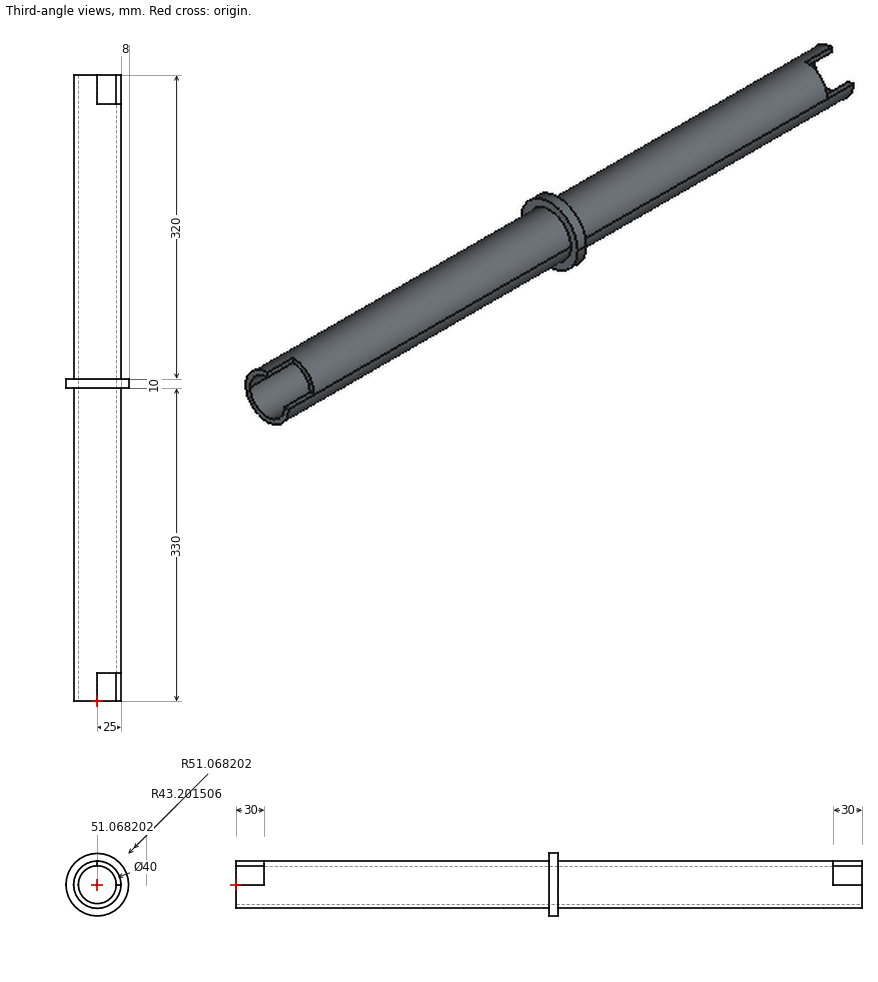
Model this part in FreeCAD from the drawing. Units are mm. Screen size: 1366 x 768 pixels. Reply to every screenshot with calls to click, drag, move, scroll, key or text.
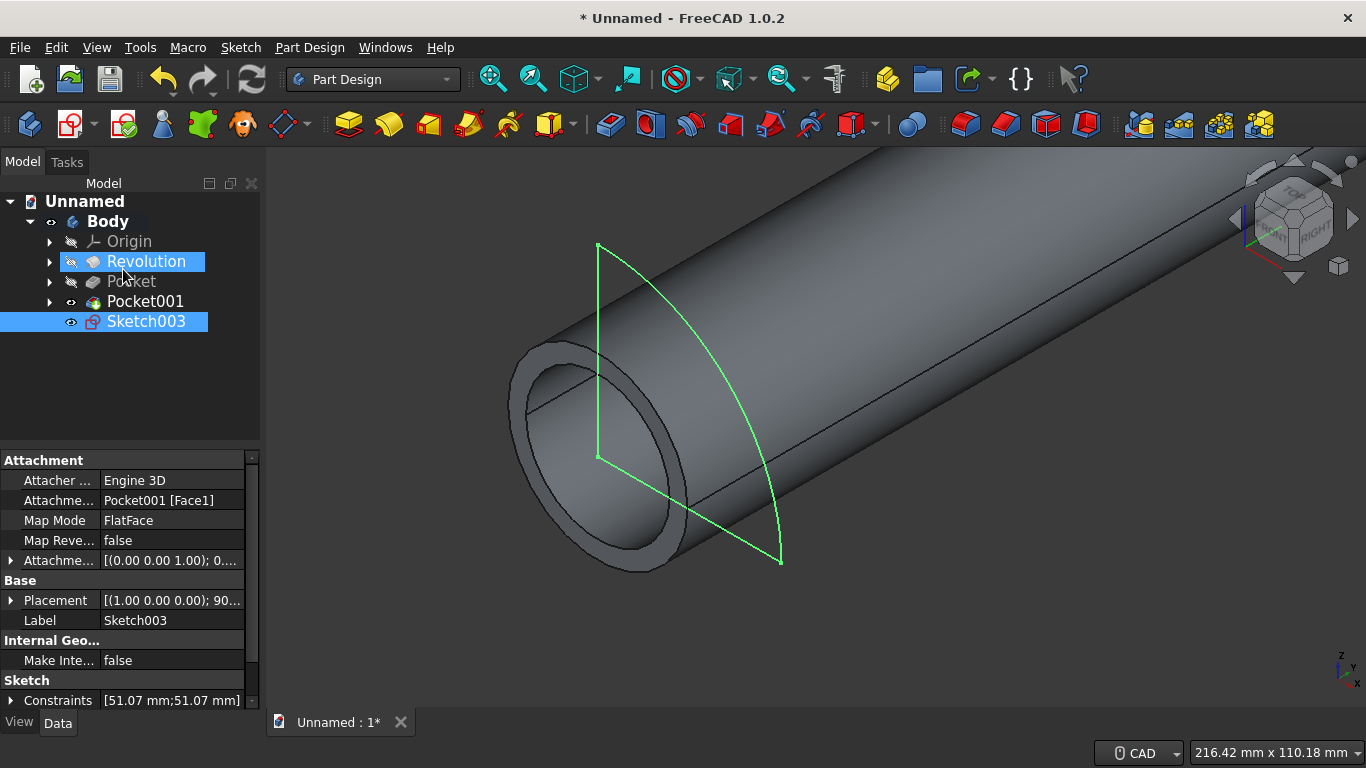
click(612, 124)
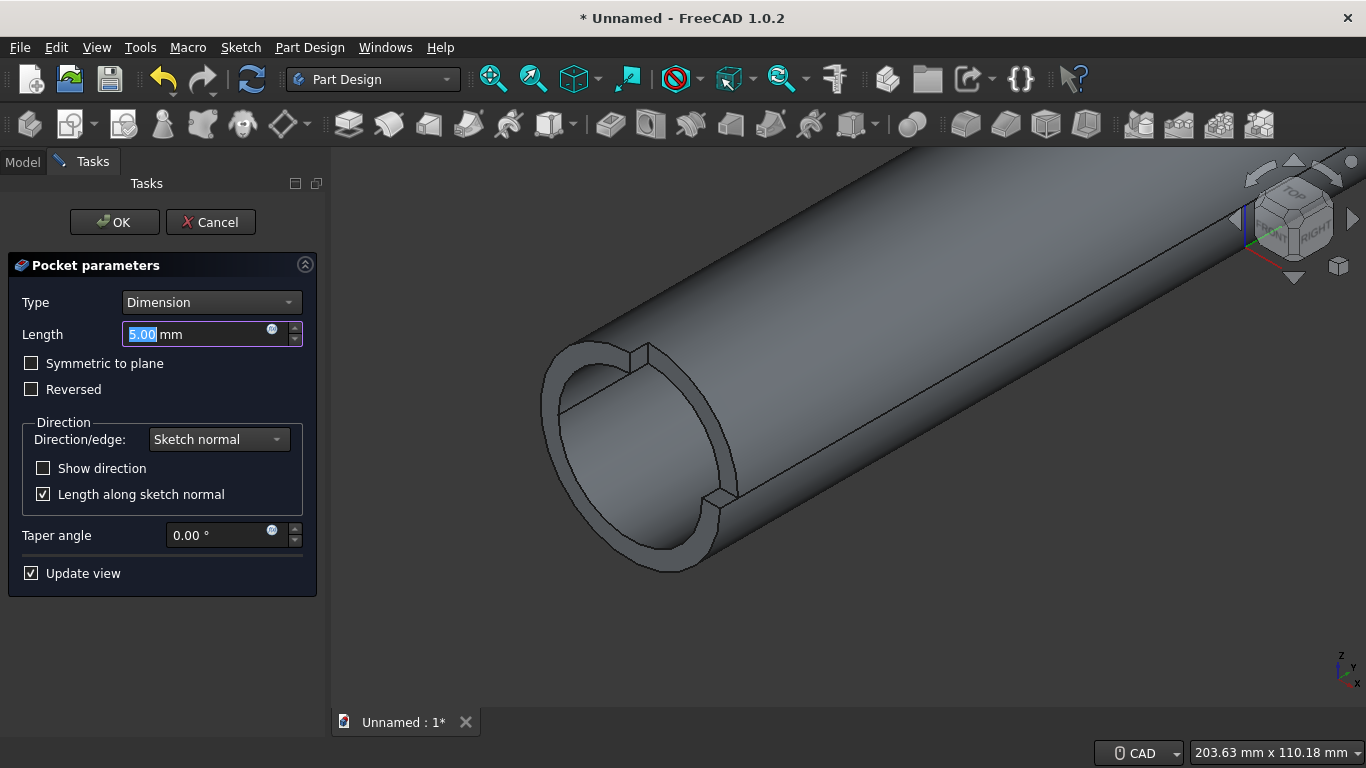
text(30)
key(Tab)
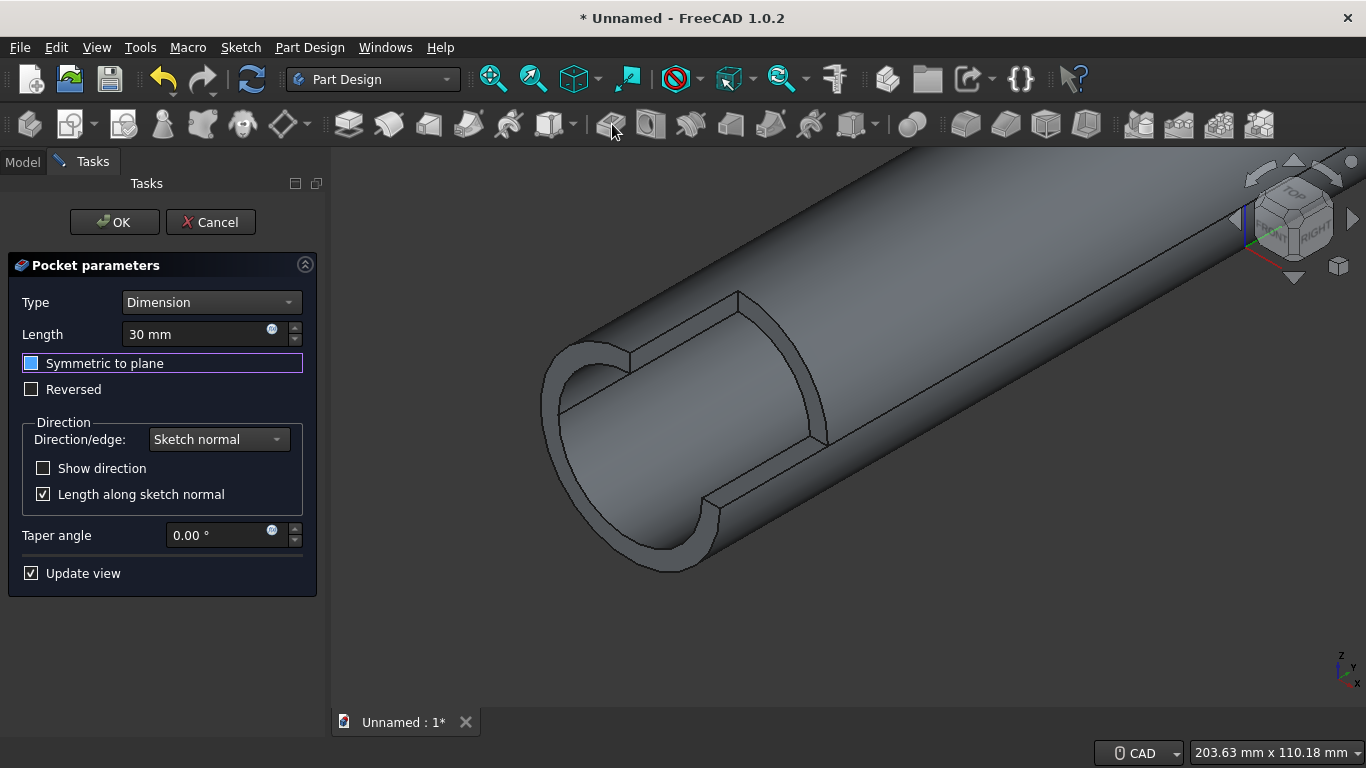
click(115, 222)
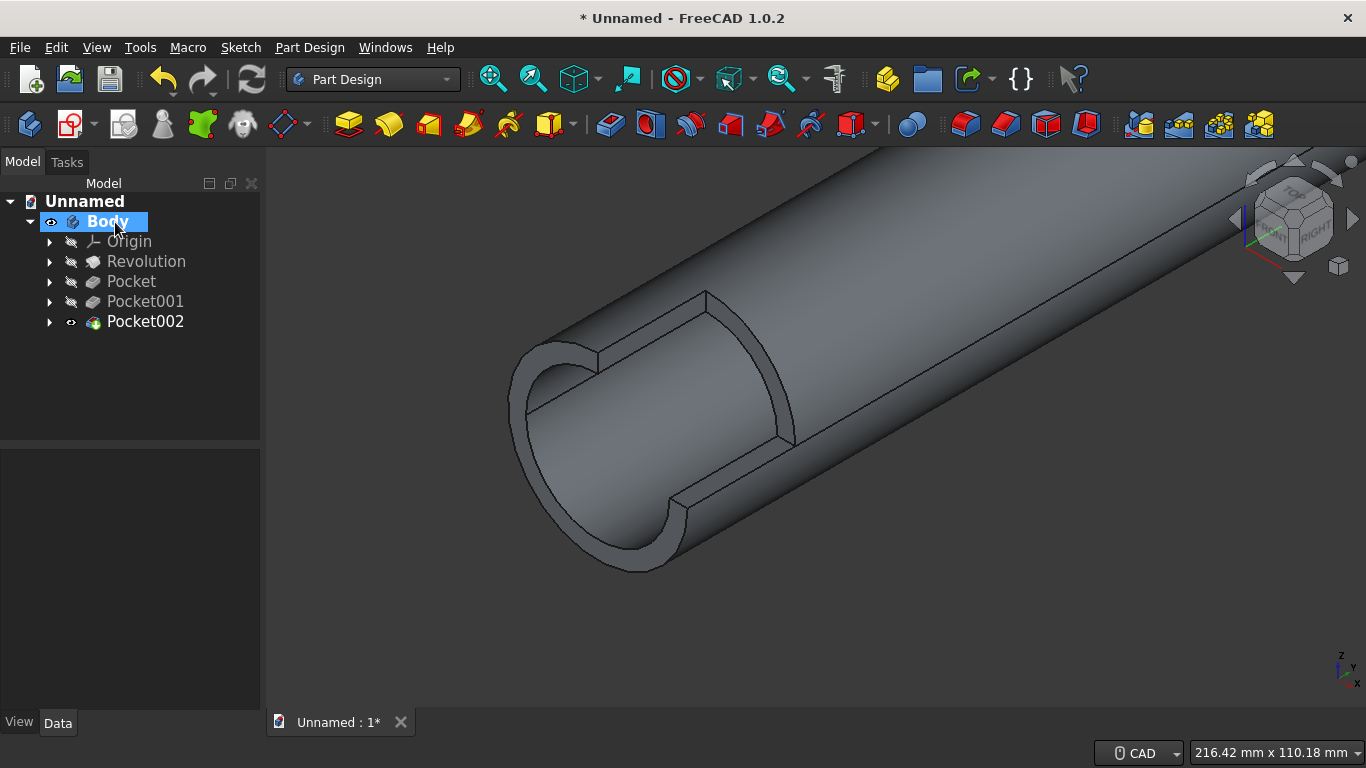
click(494, 80)